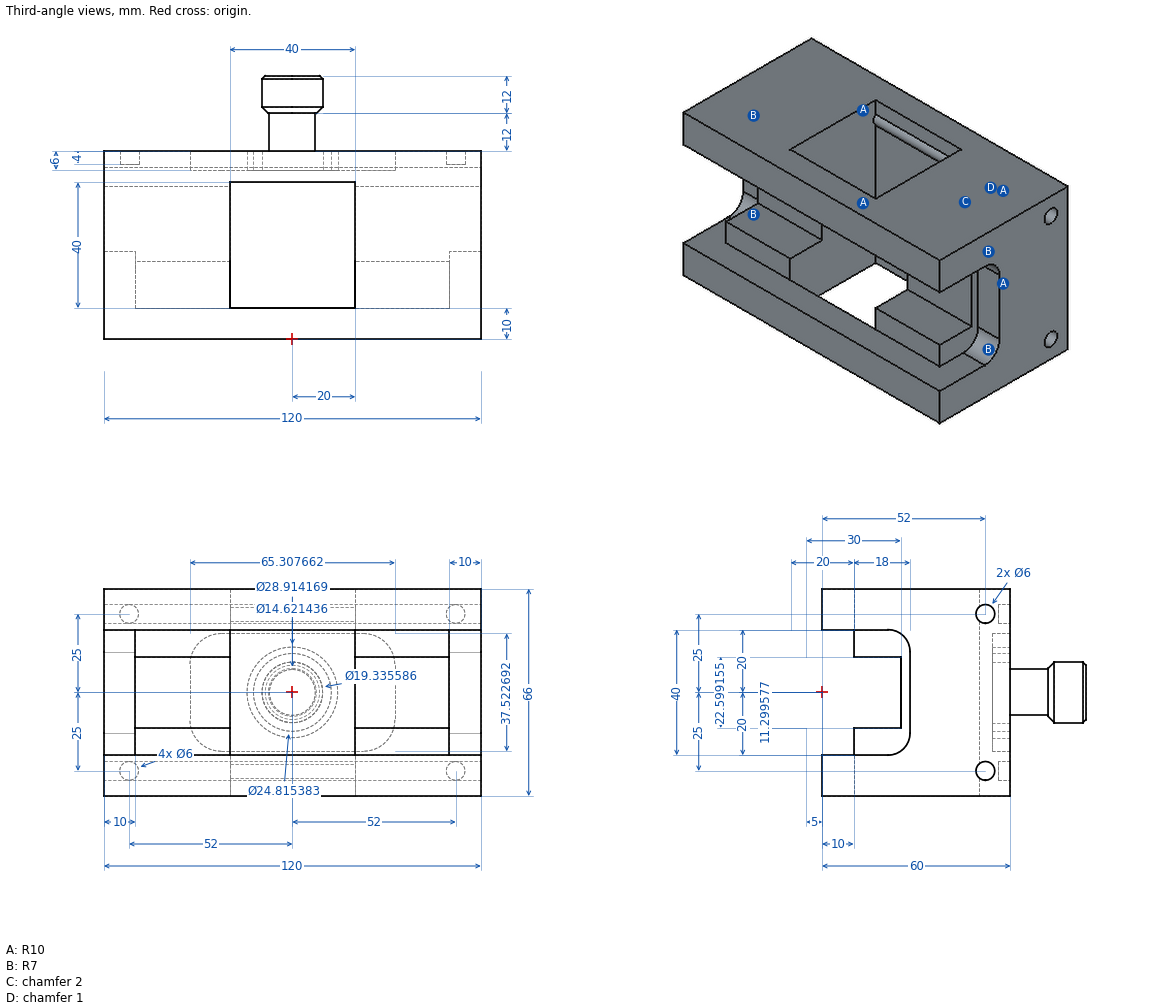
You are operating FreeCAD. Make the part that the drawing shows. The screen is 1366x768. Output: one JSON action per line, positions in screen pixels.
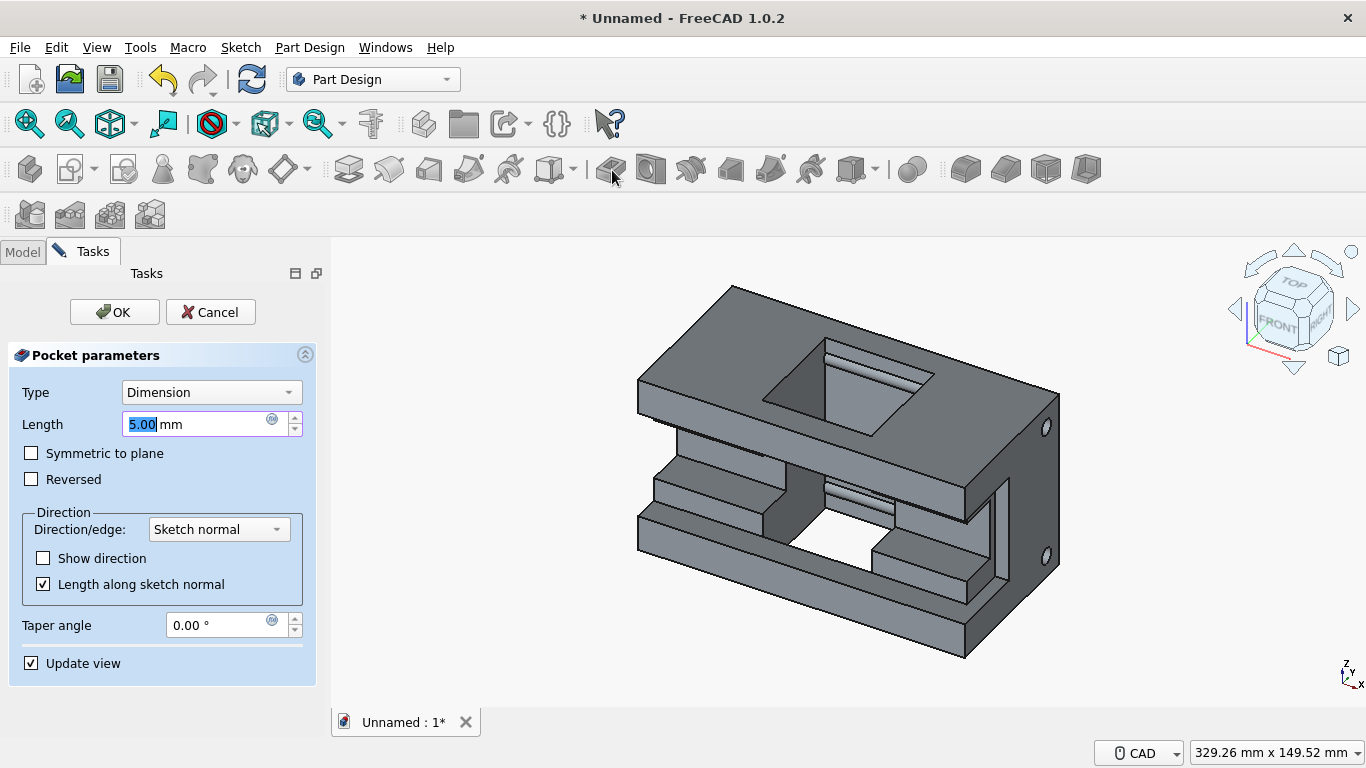
{"action": "type", "text": "10"}
{"action": "key", "text": "Tab"}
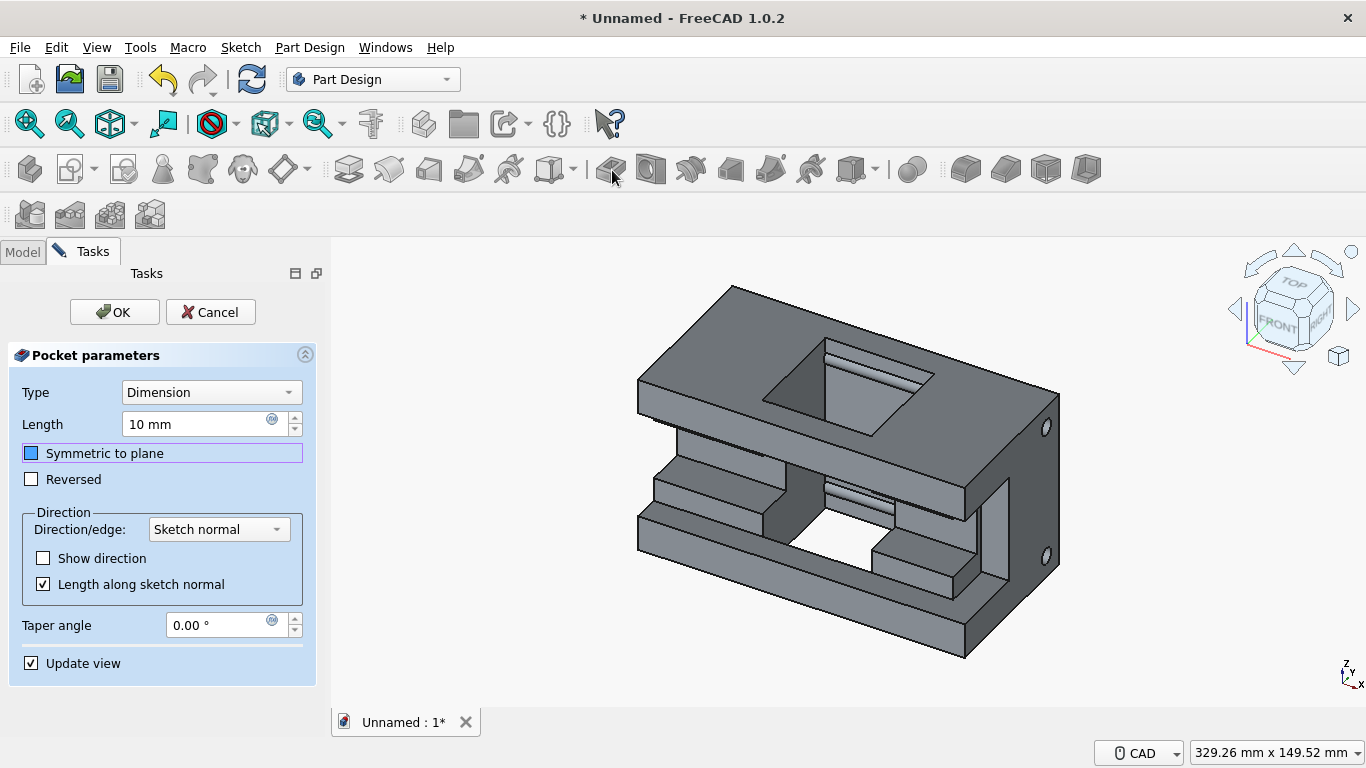
{"action": "left_click", "coordinate": [115, 312]}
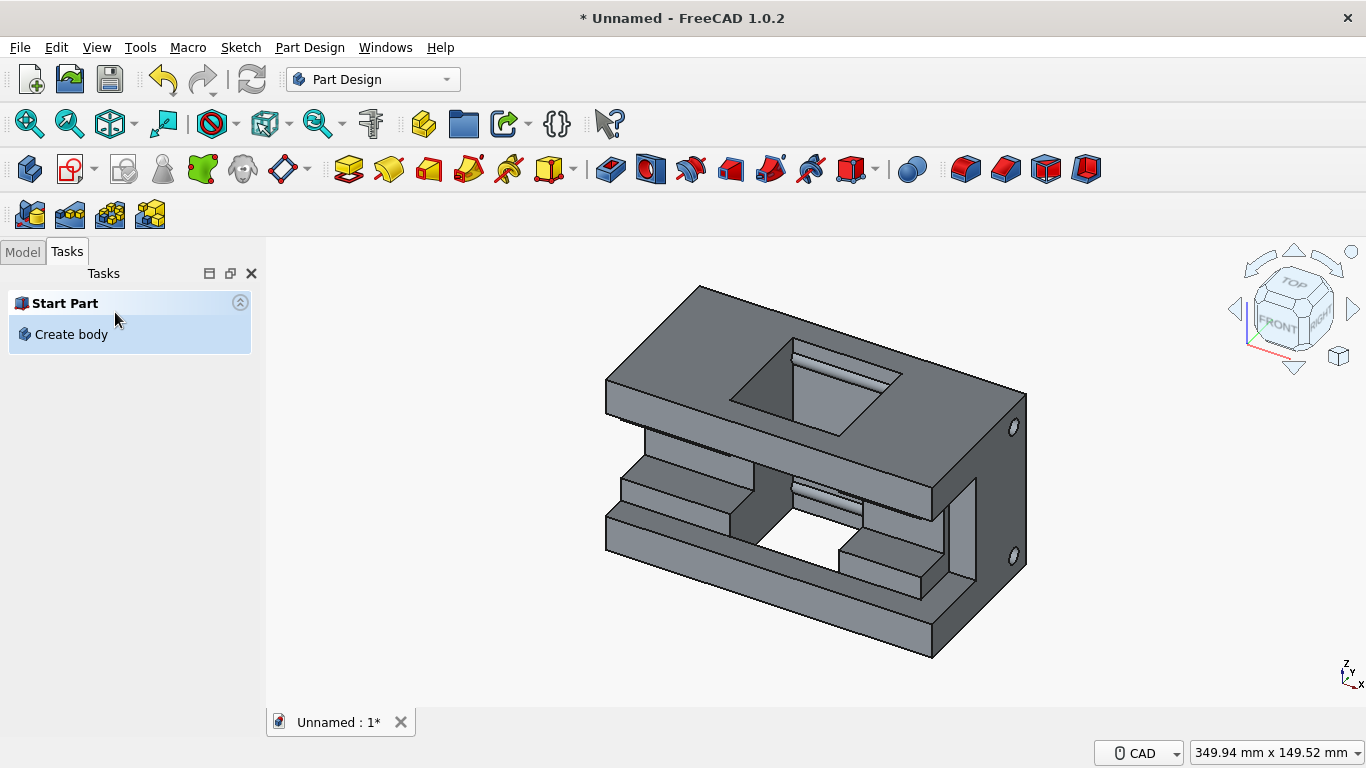
{"action": "key", "text": "6"}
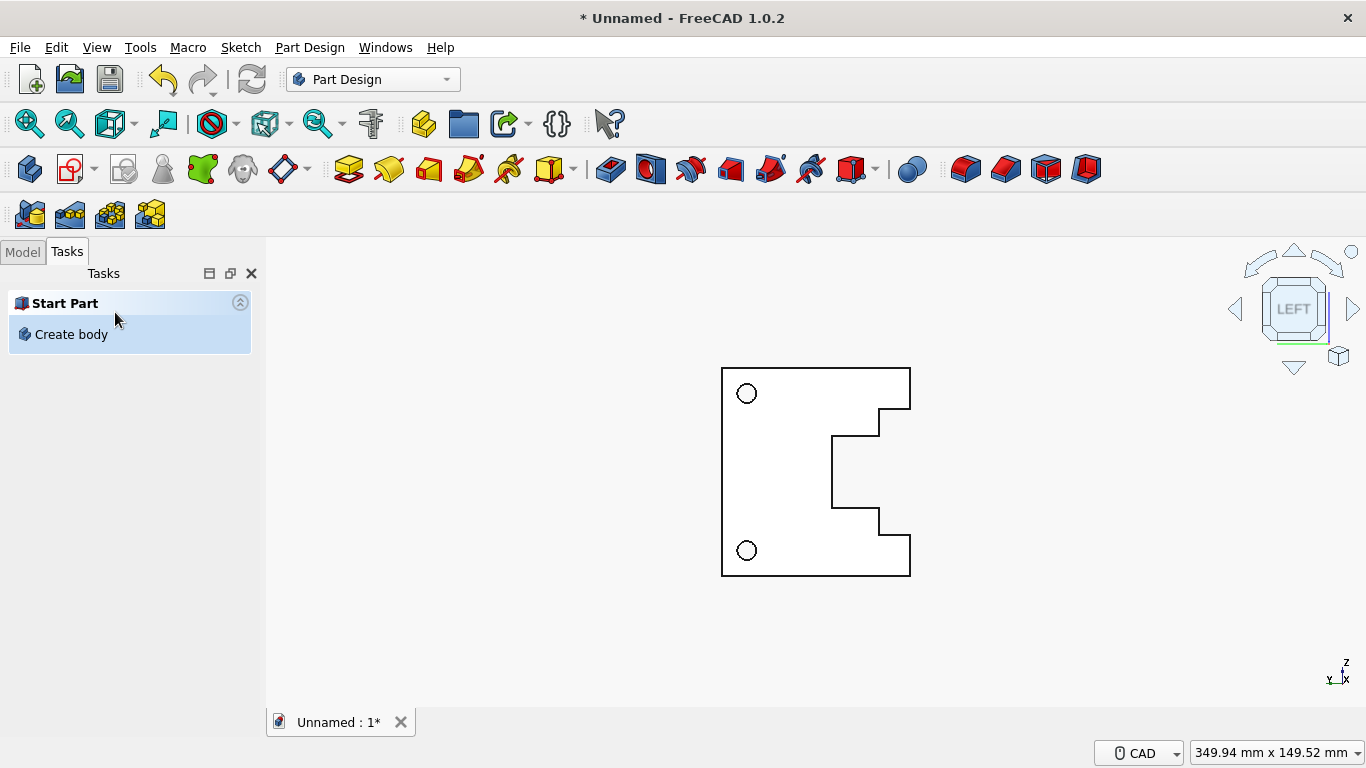
{"action": "left_click", "coordinate": [30, 124]}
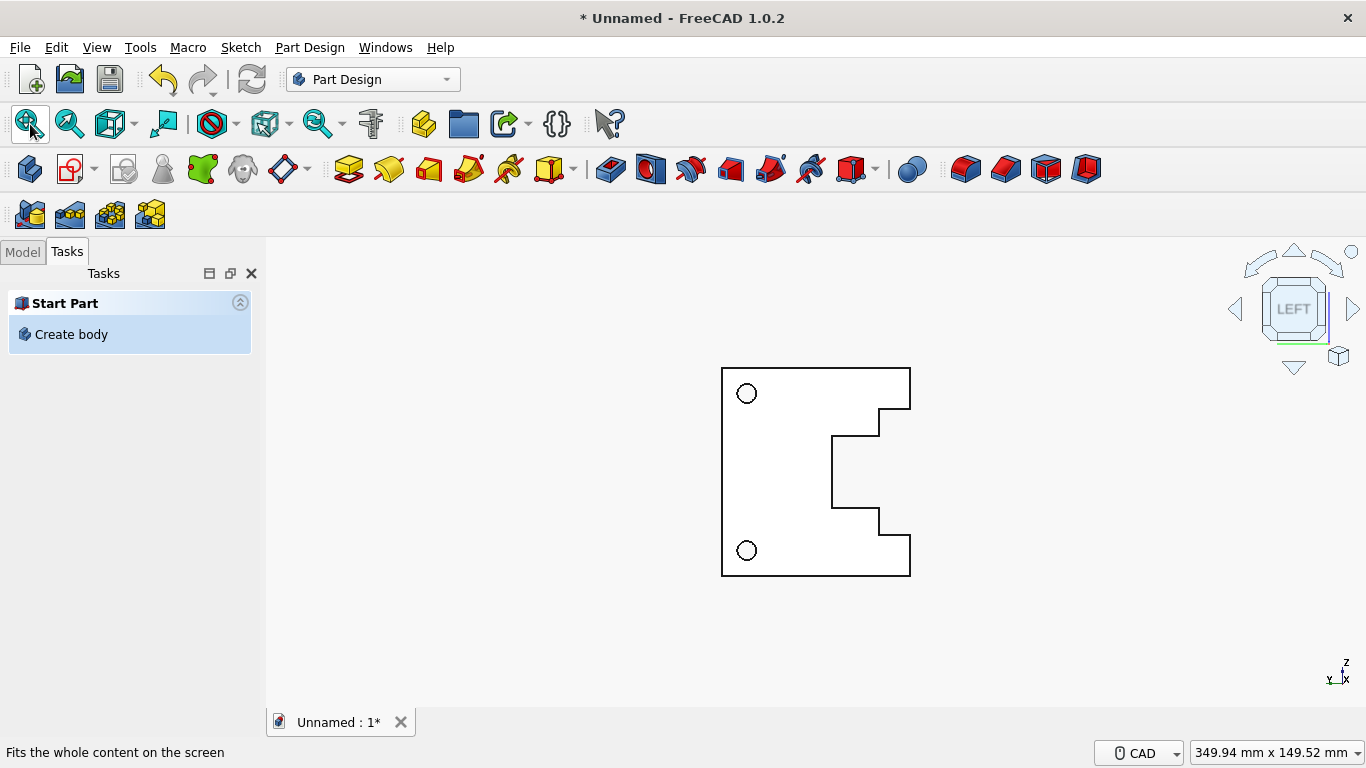
{"action": "left_click", "coordinate": [789, 441]}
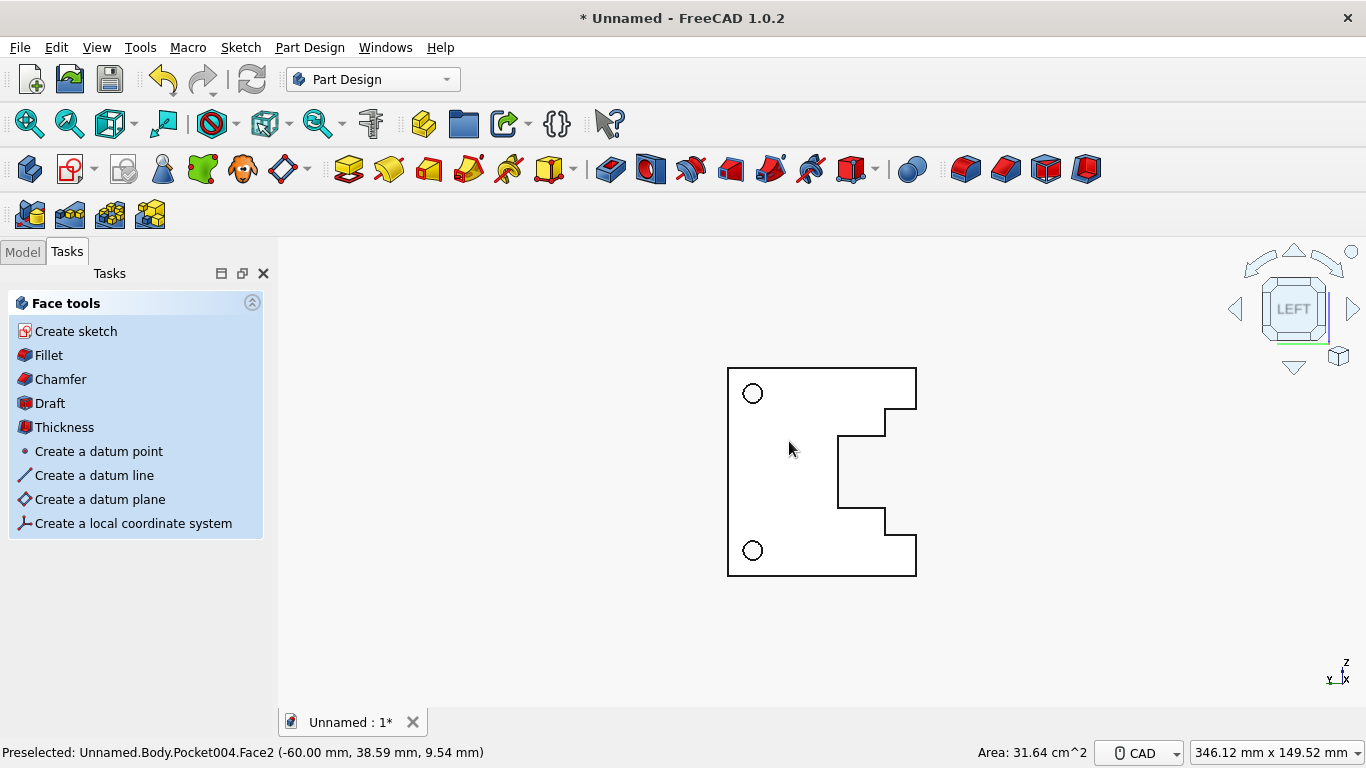
{"action": "left_click", "coordinate": [70, 170]}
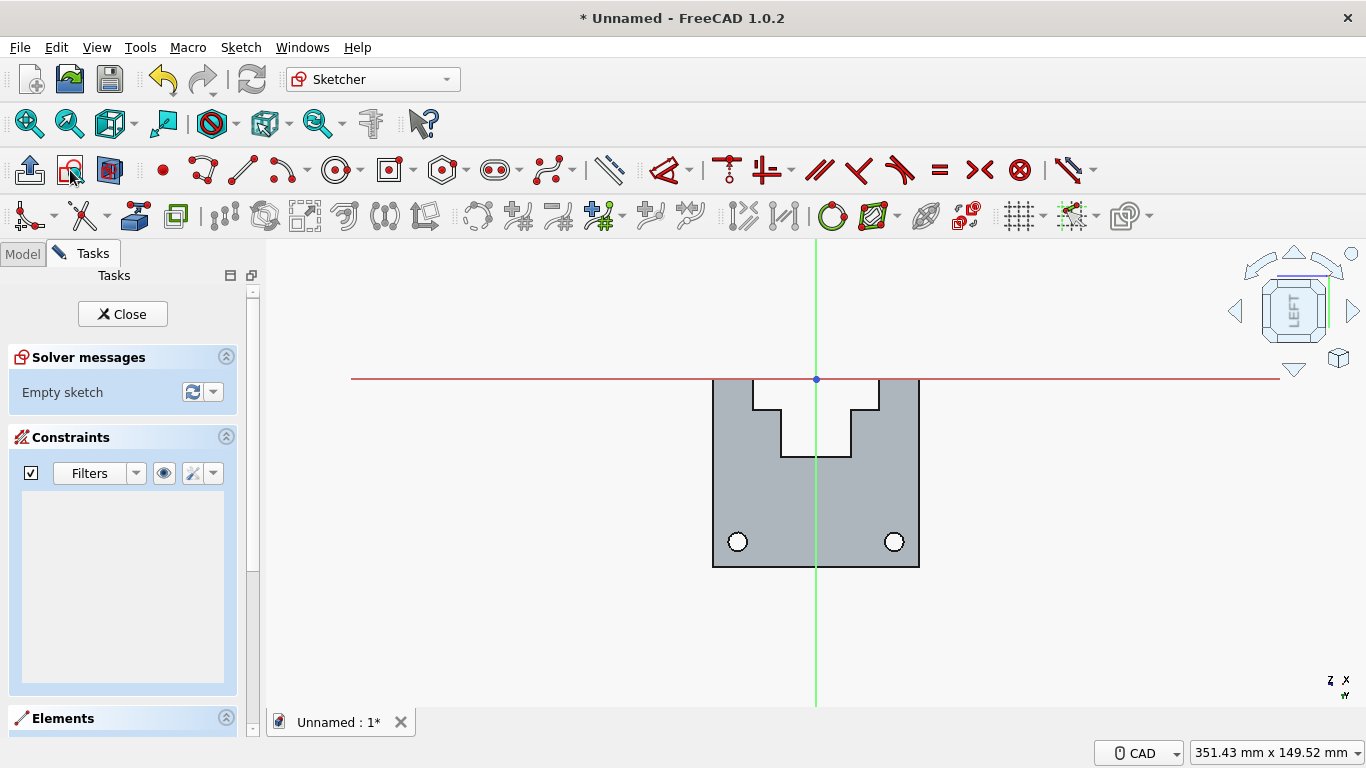
{"action": "scroll", "coordinate": [846, 401], "scroll_direction": "up", "scroll_amount": 6}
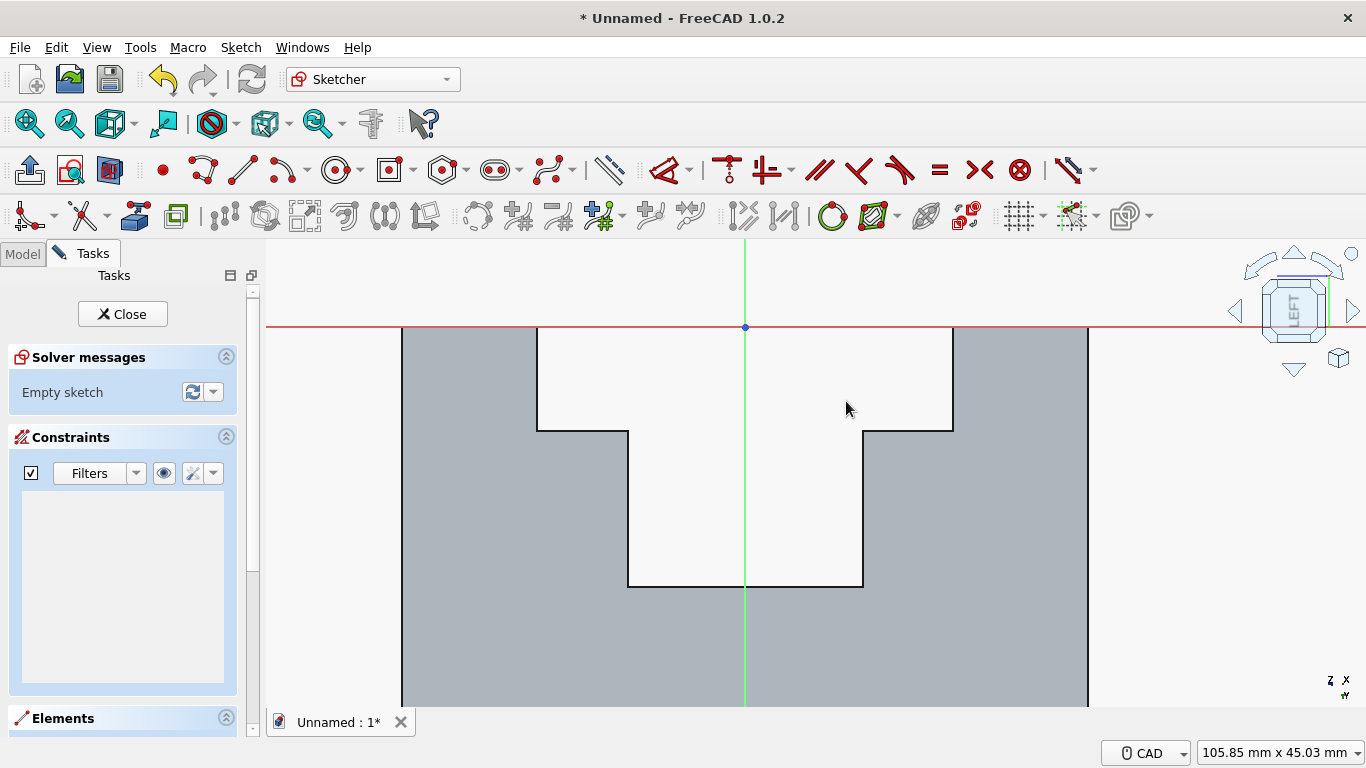
{"action": "key", "text": "g r"}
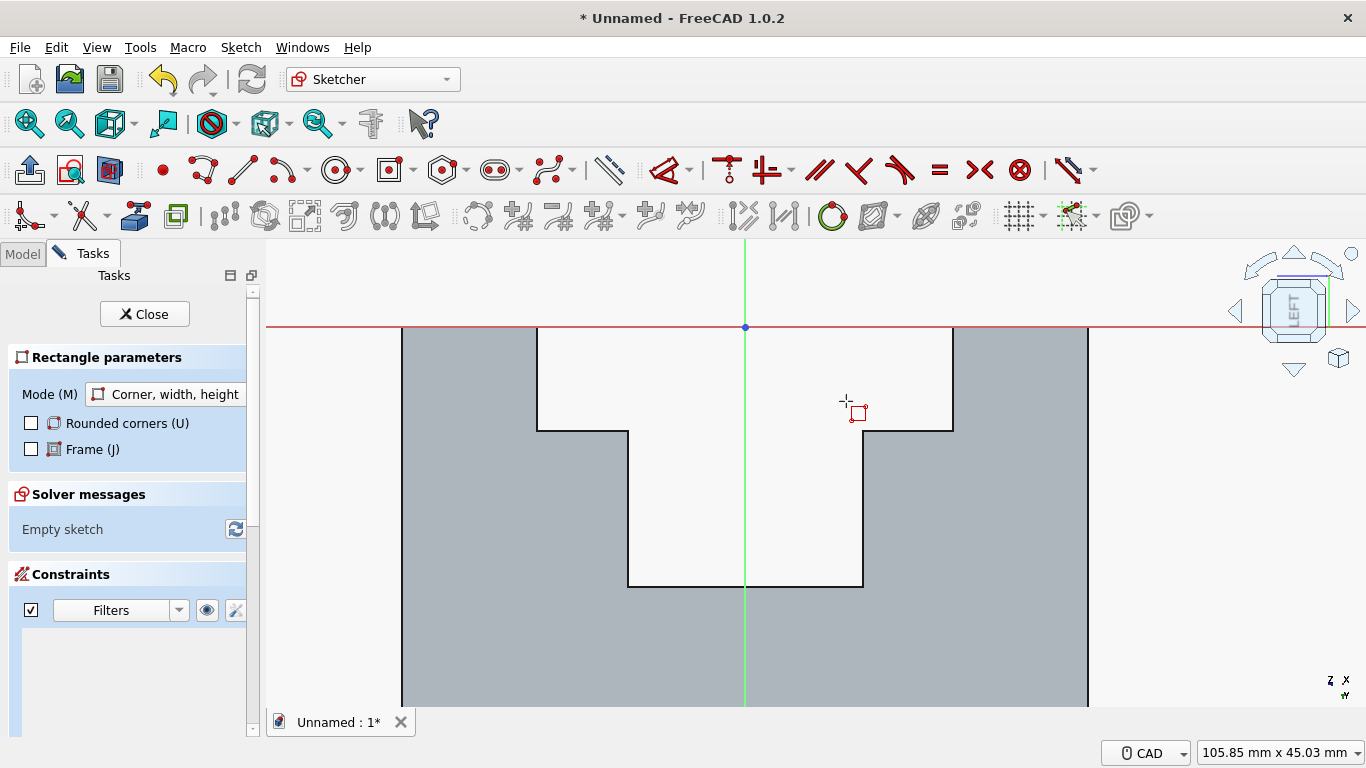
{"action": "left_click", "coordinate": [537, 431]}
{"action": "mouse_move", "coordinate": [953, 618]}